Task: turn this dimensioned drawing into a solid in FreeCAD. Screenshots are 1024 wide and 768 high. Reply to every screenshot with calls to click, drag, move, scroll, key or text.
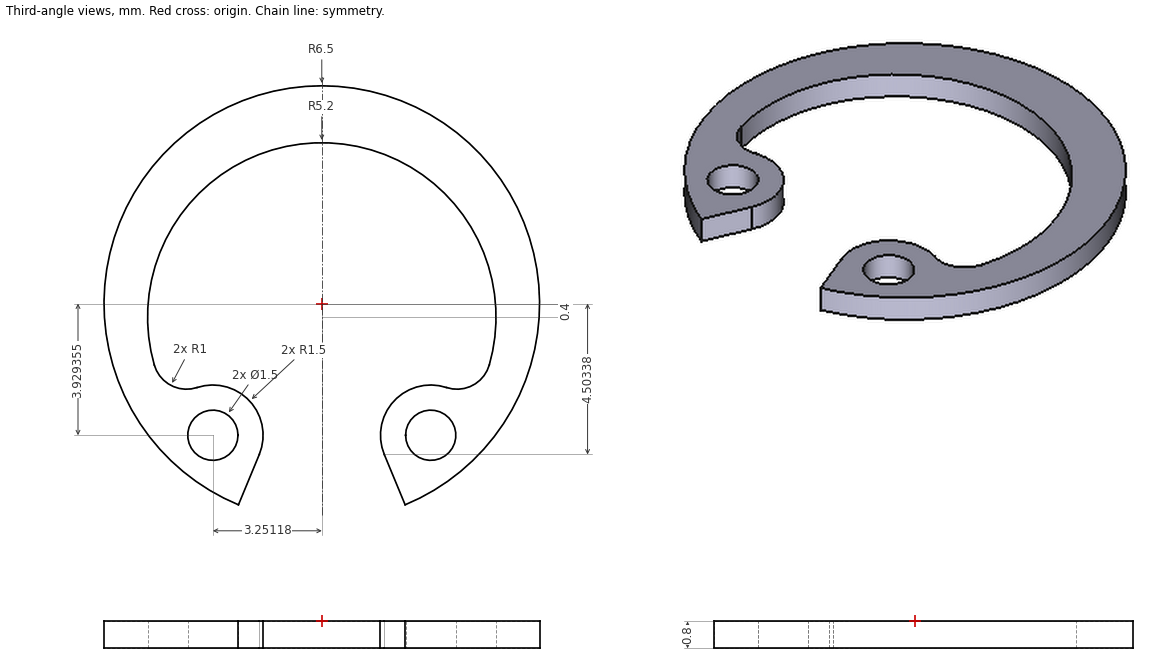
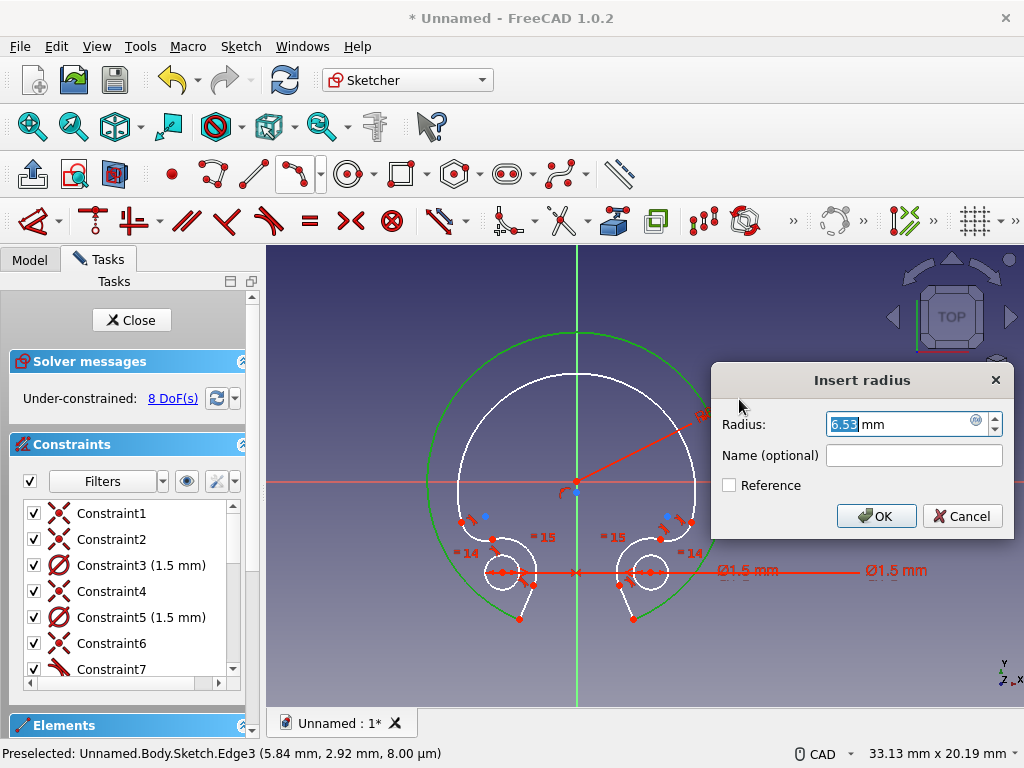
text(6.5)
key(Return)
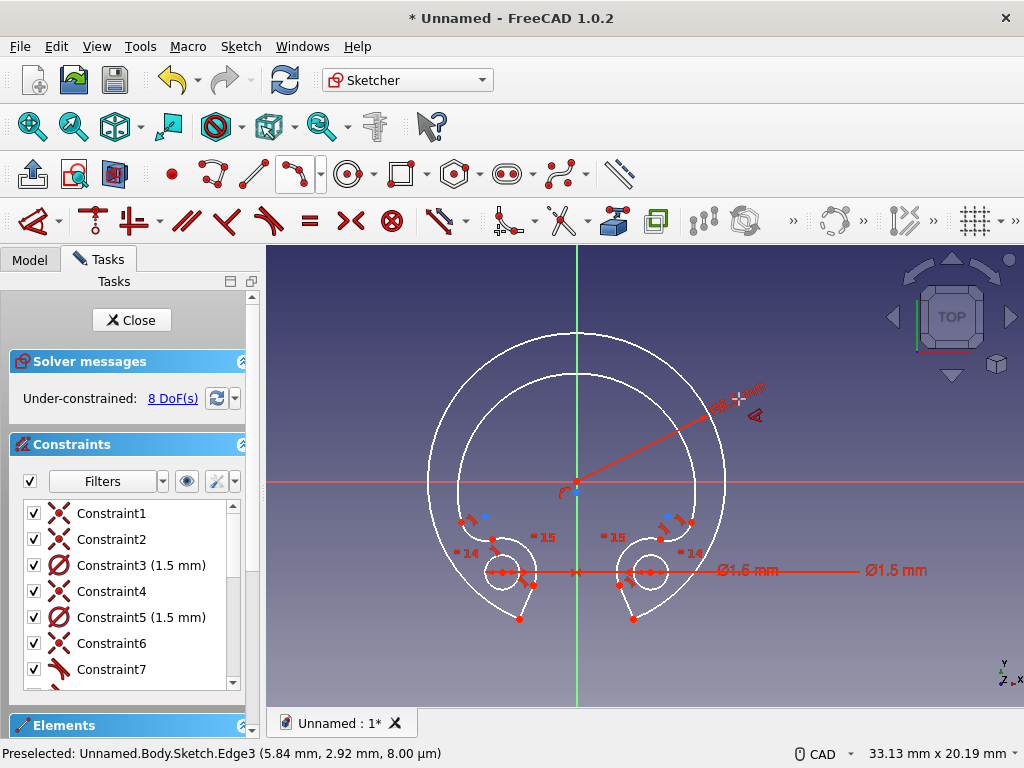
click(535, 563)
click(549, 526)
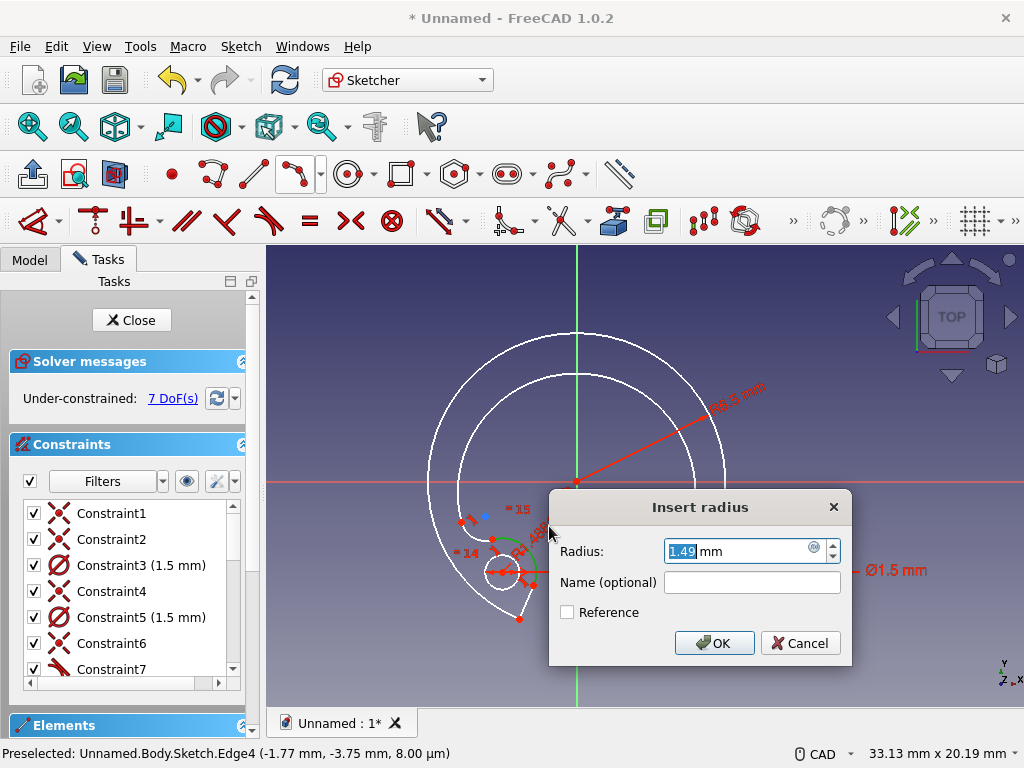
text(1.5)
key(Return)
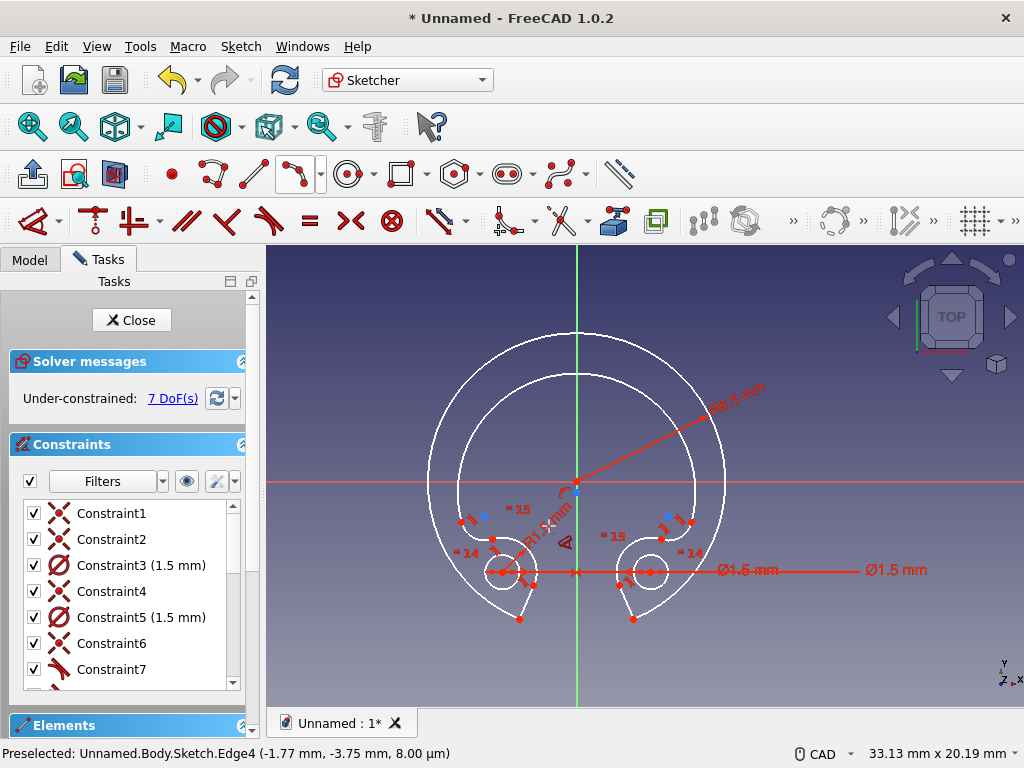
scroll(467, 533, up, 3)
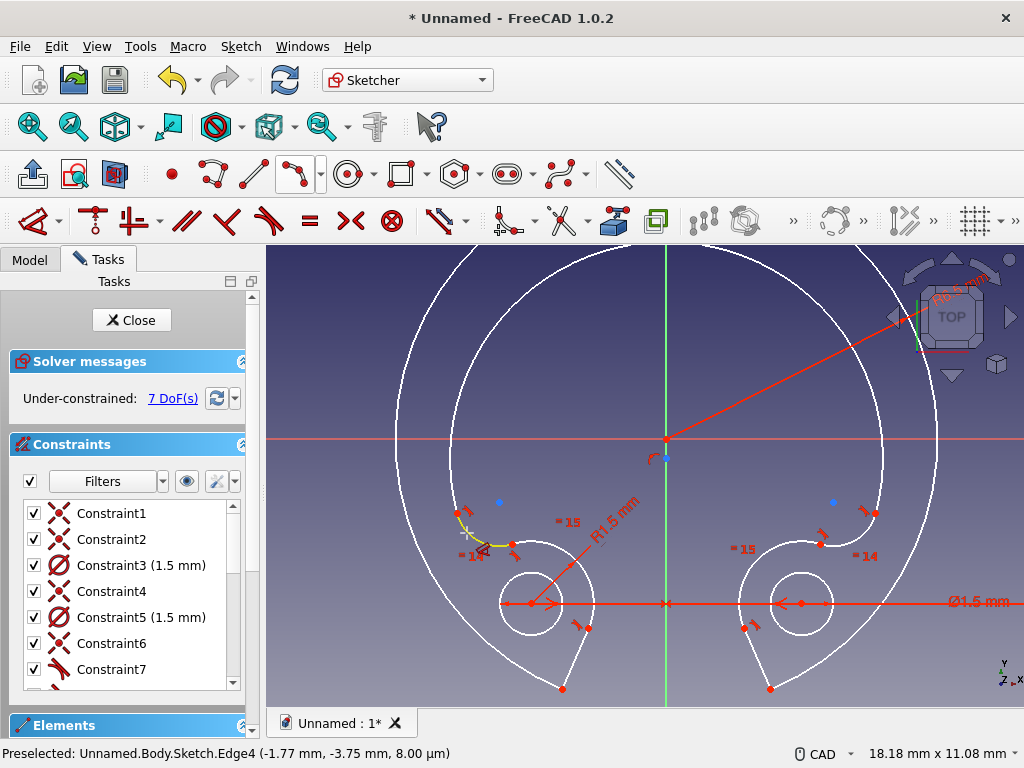
click(467, 532)
click(443, 554)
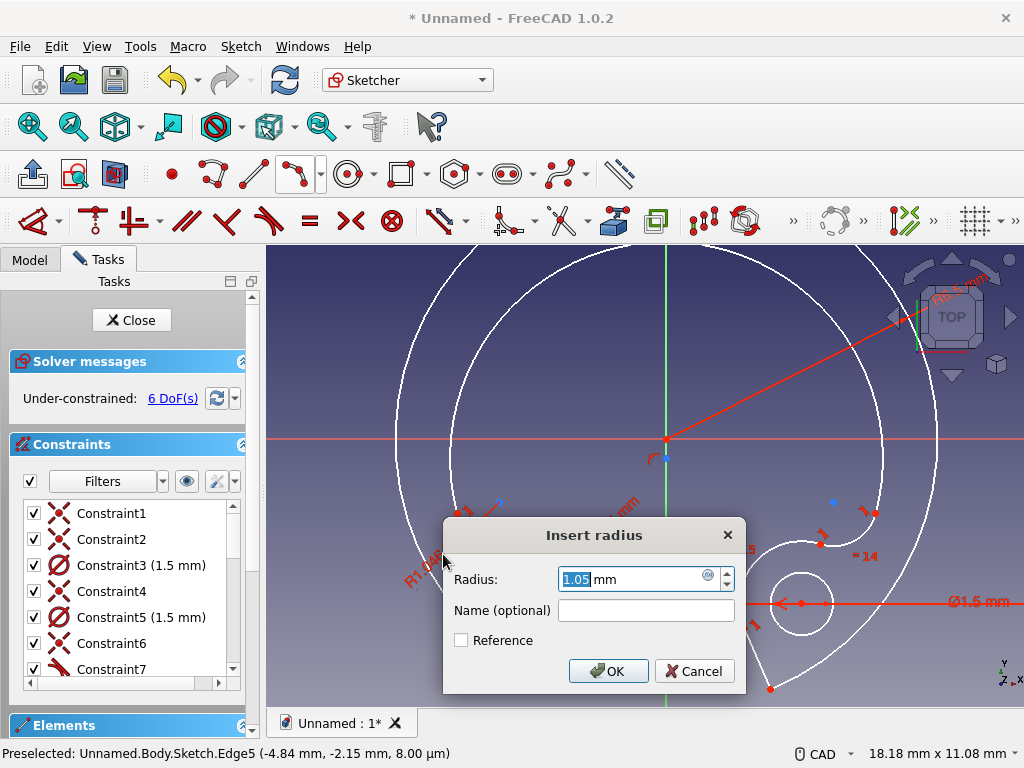
text(1)
key(Return)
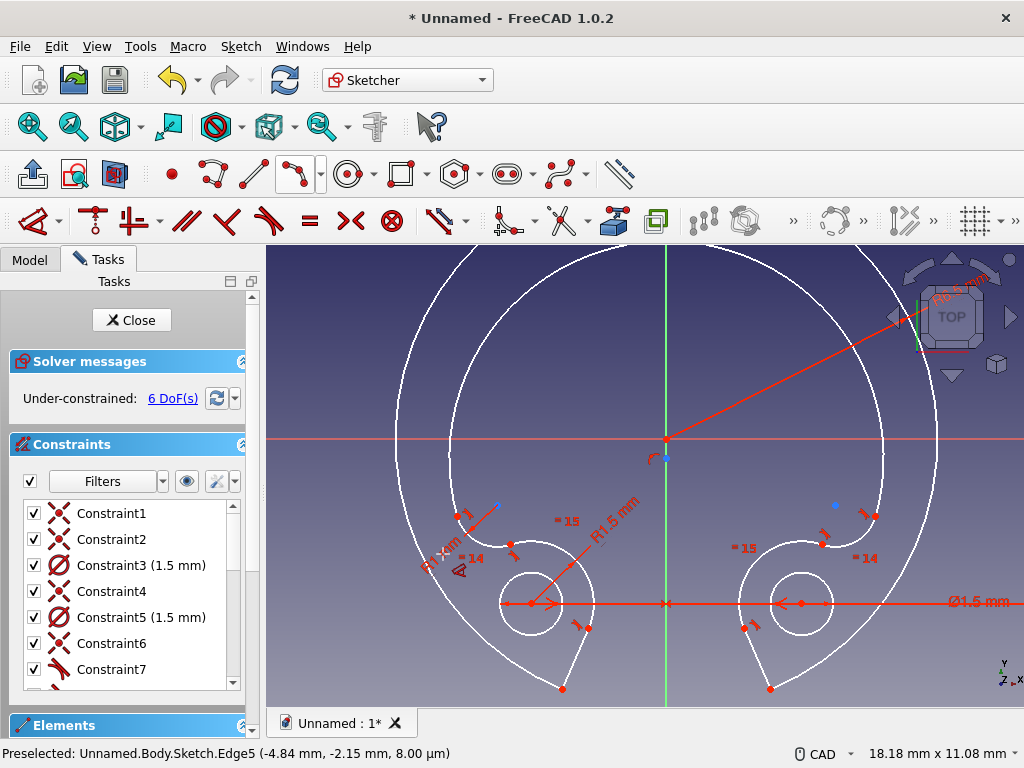
click(812, 298)
click(834, 274)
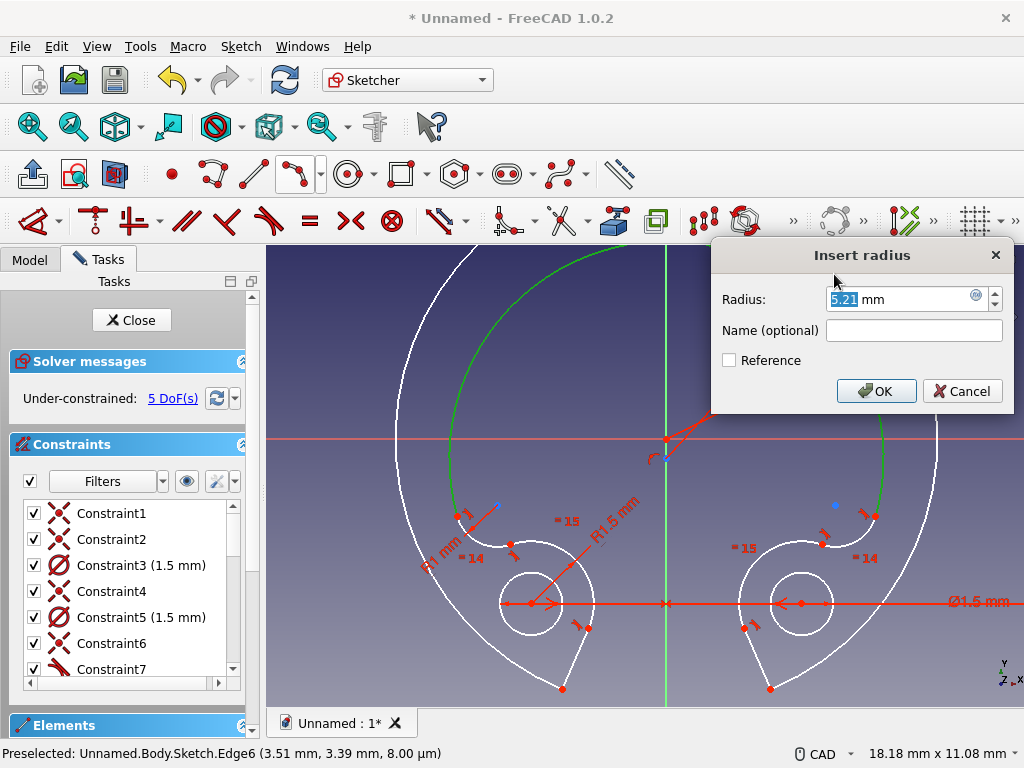
text(5.2)
key(Return)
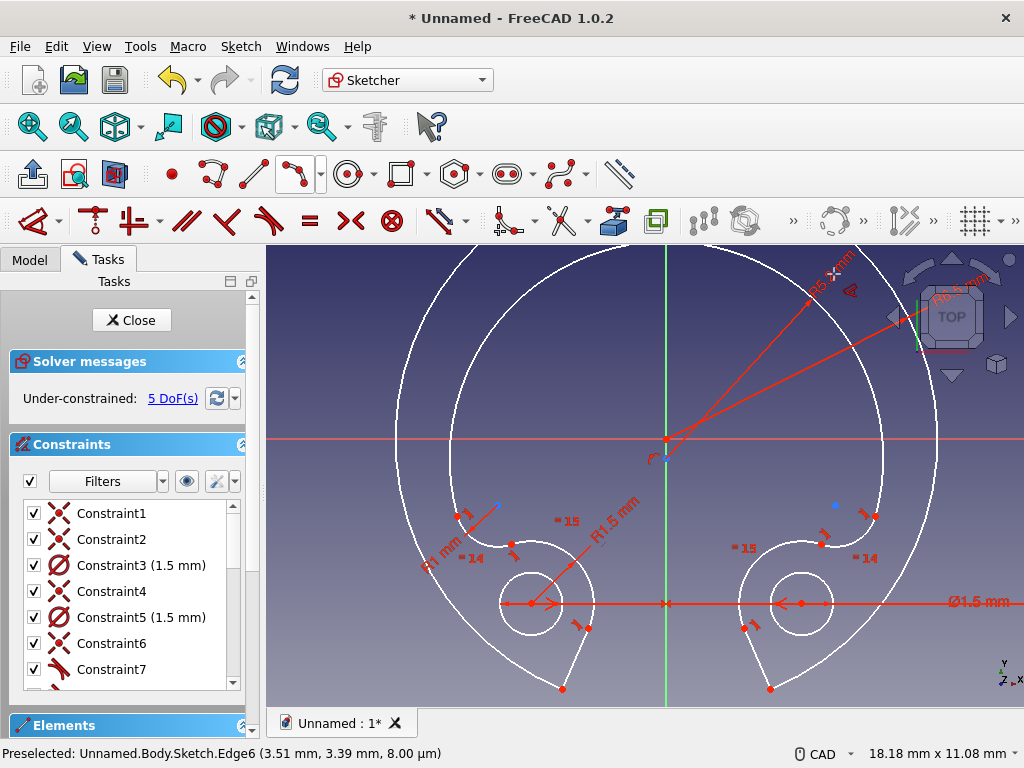
scroll(666, 458, up, 5)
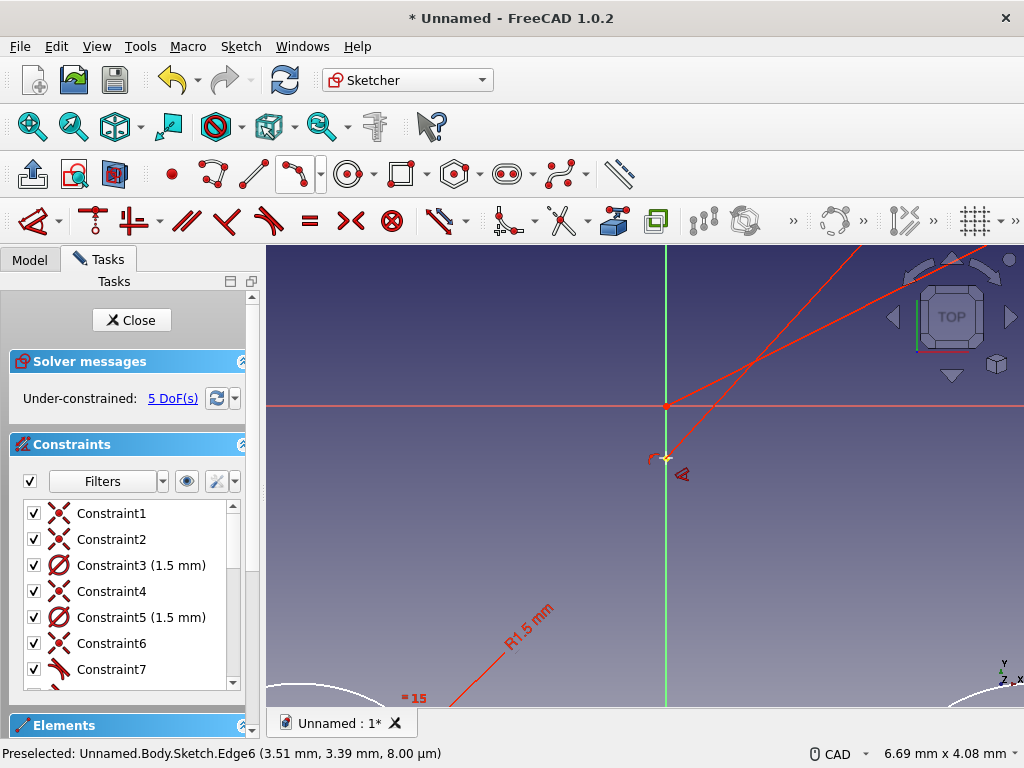
click(666, 458)
click(700, 432)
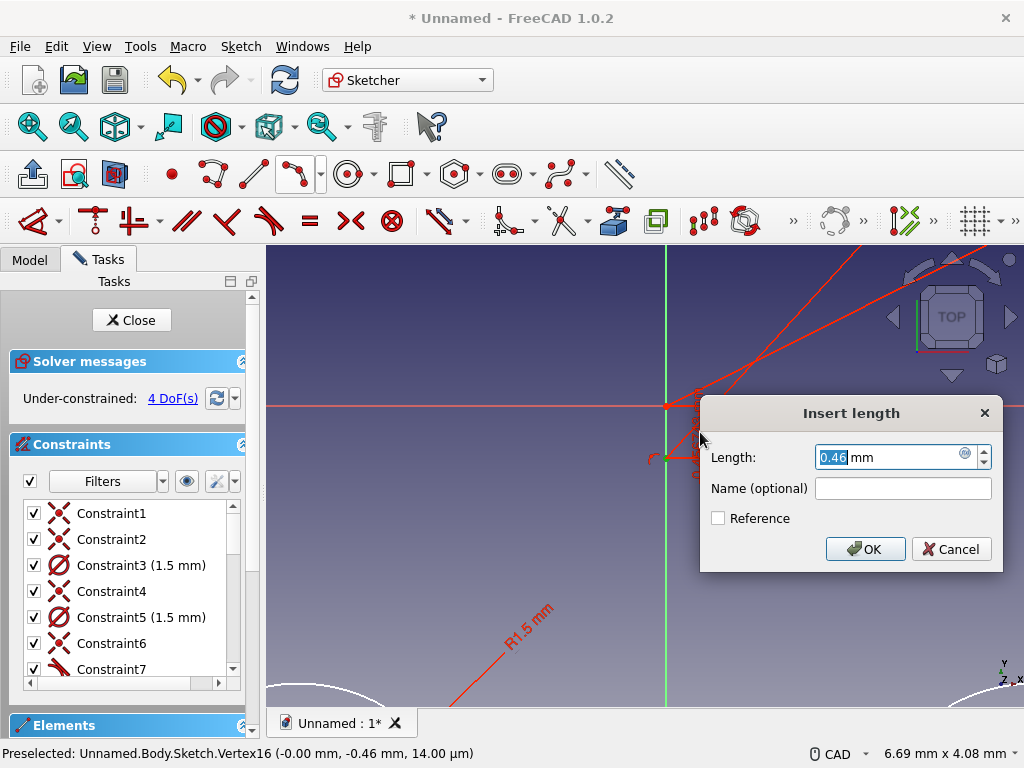
text(0.4)
key(Return)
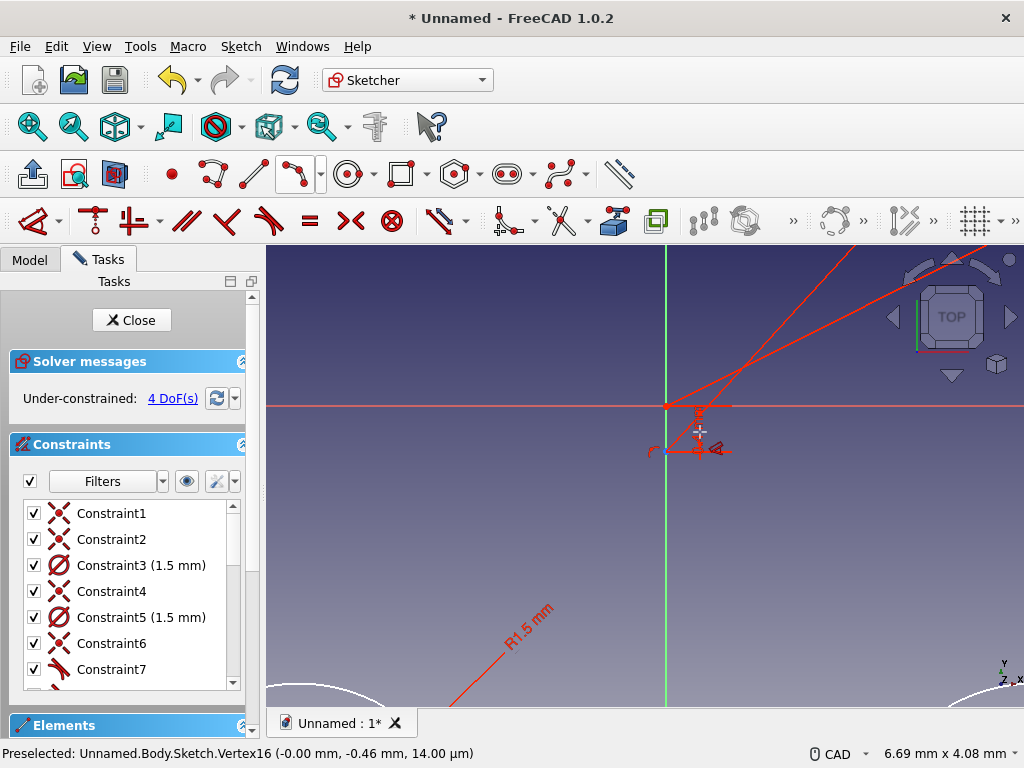
scroll(554, 501, down, 8)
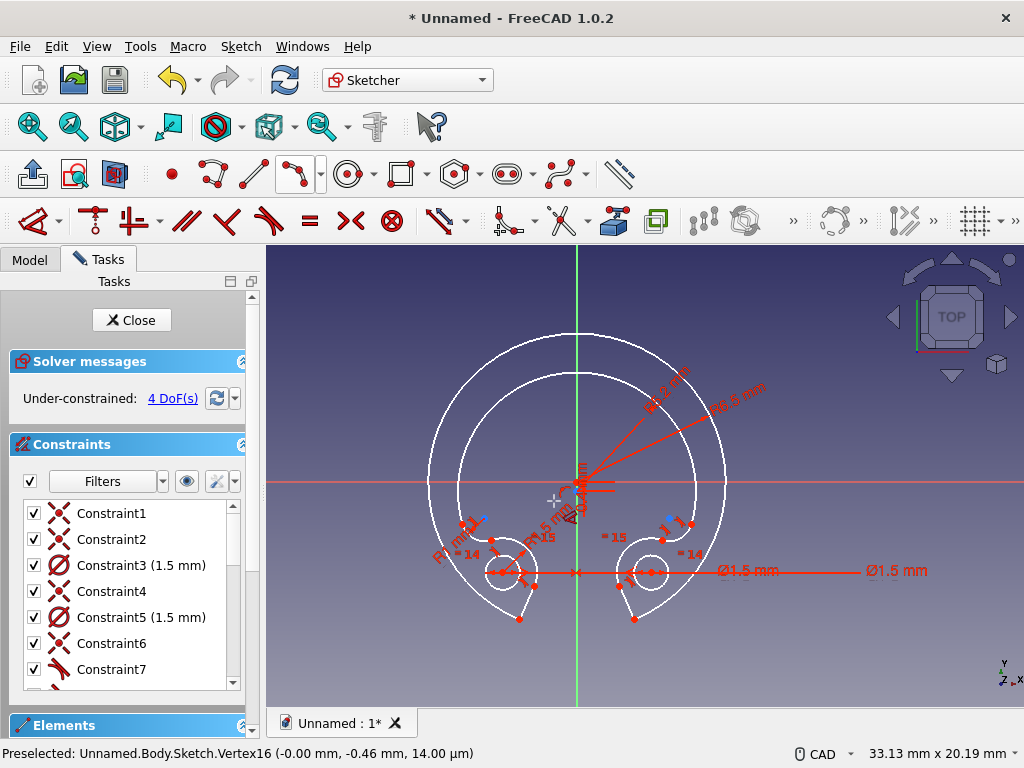
click(503, 573)
click(540, 607)